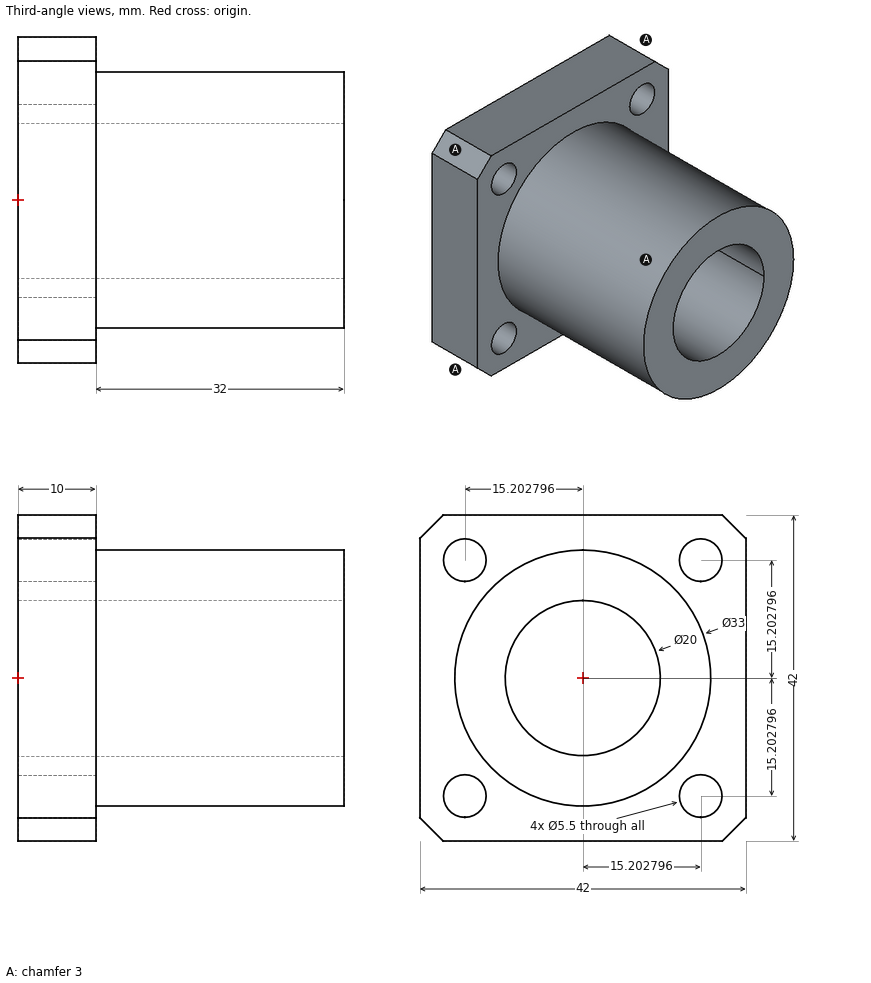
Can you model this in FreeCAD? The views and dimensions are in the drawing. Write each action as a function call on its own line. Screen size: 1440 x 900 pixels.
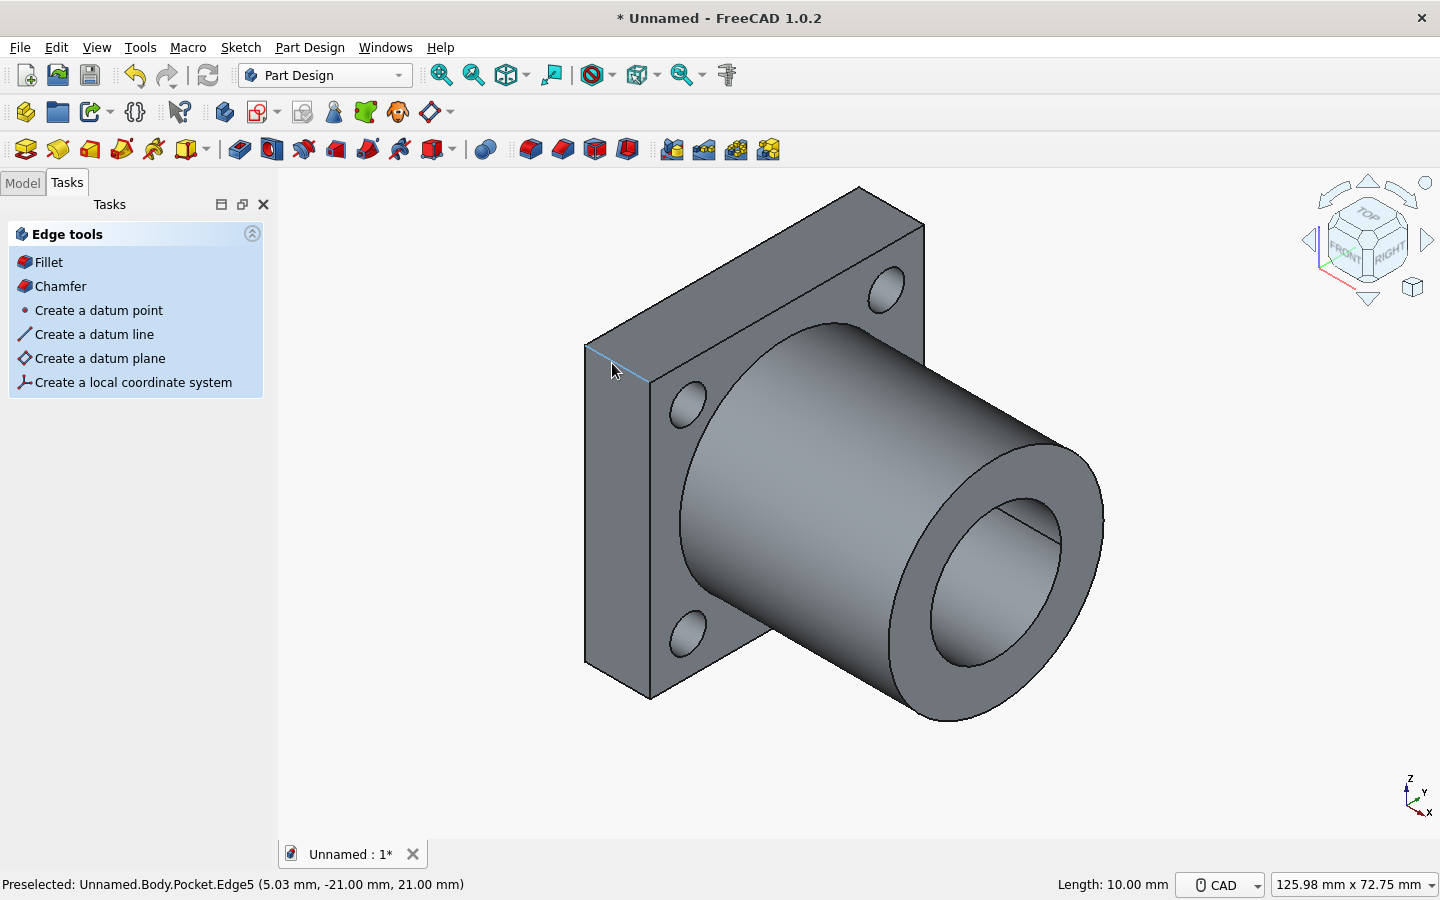
key(2)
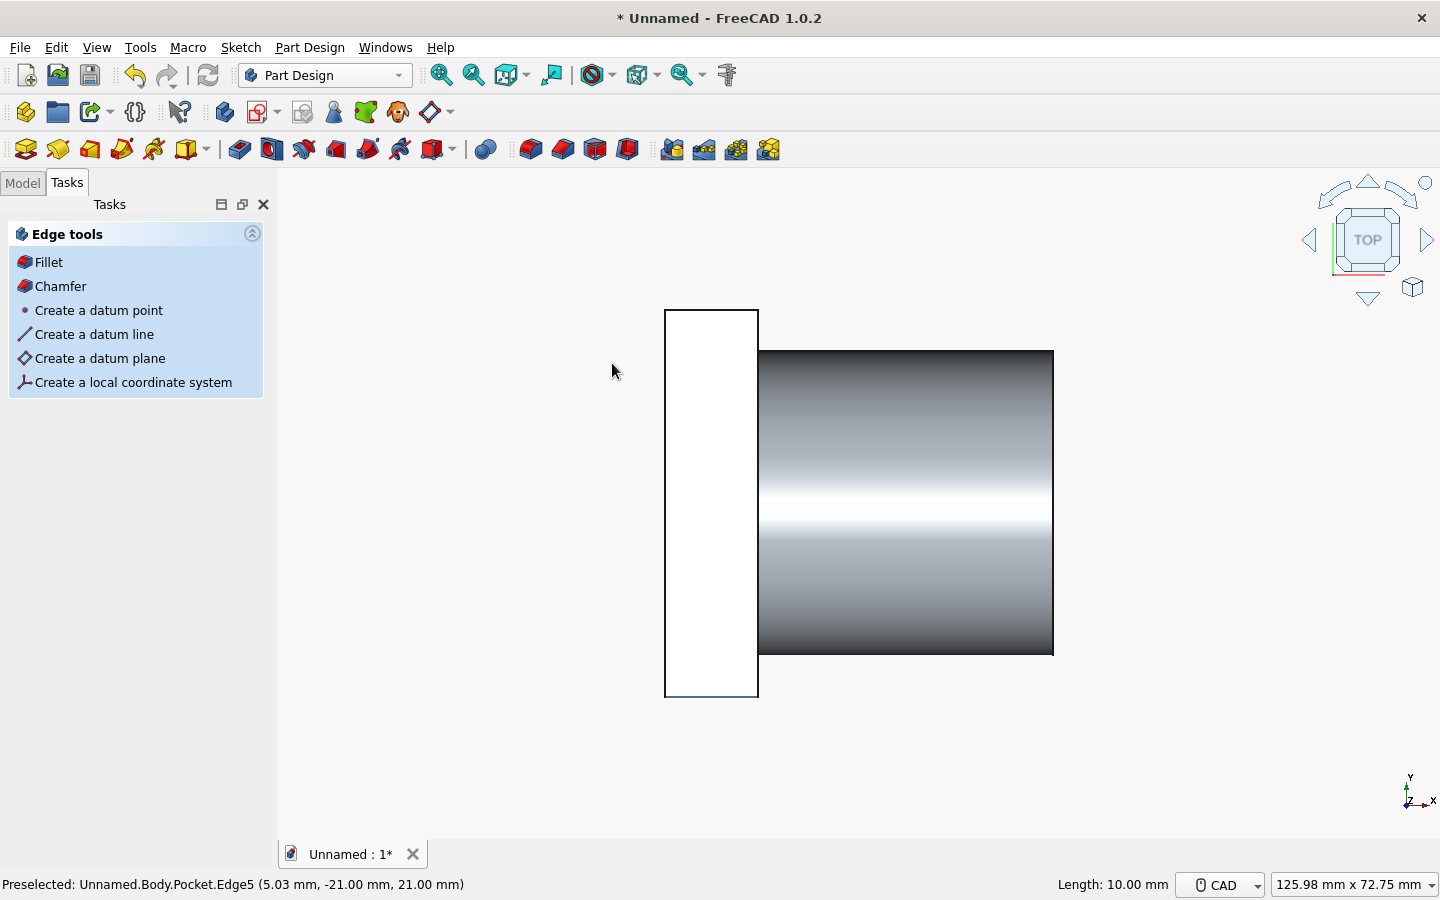
click(711, 309, ctrl)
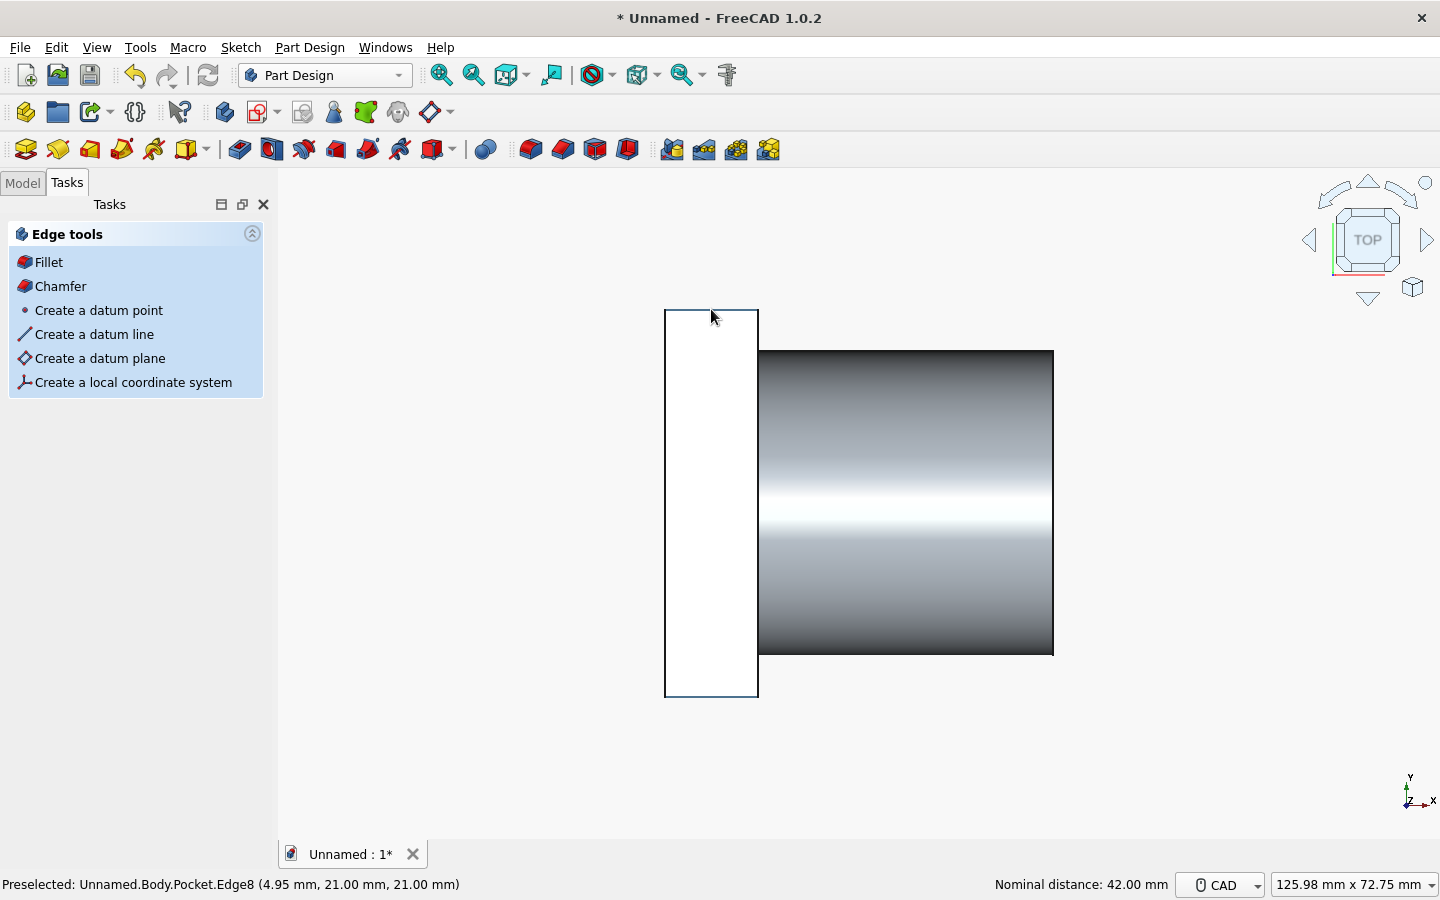
key(1)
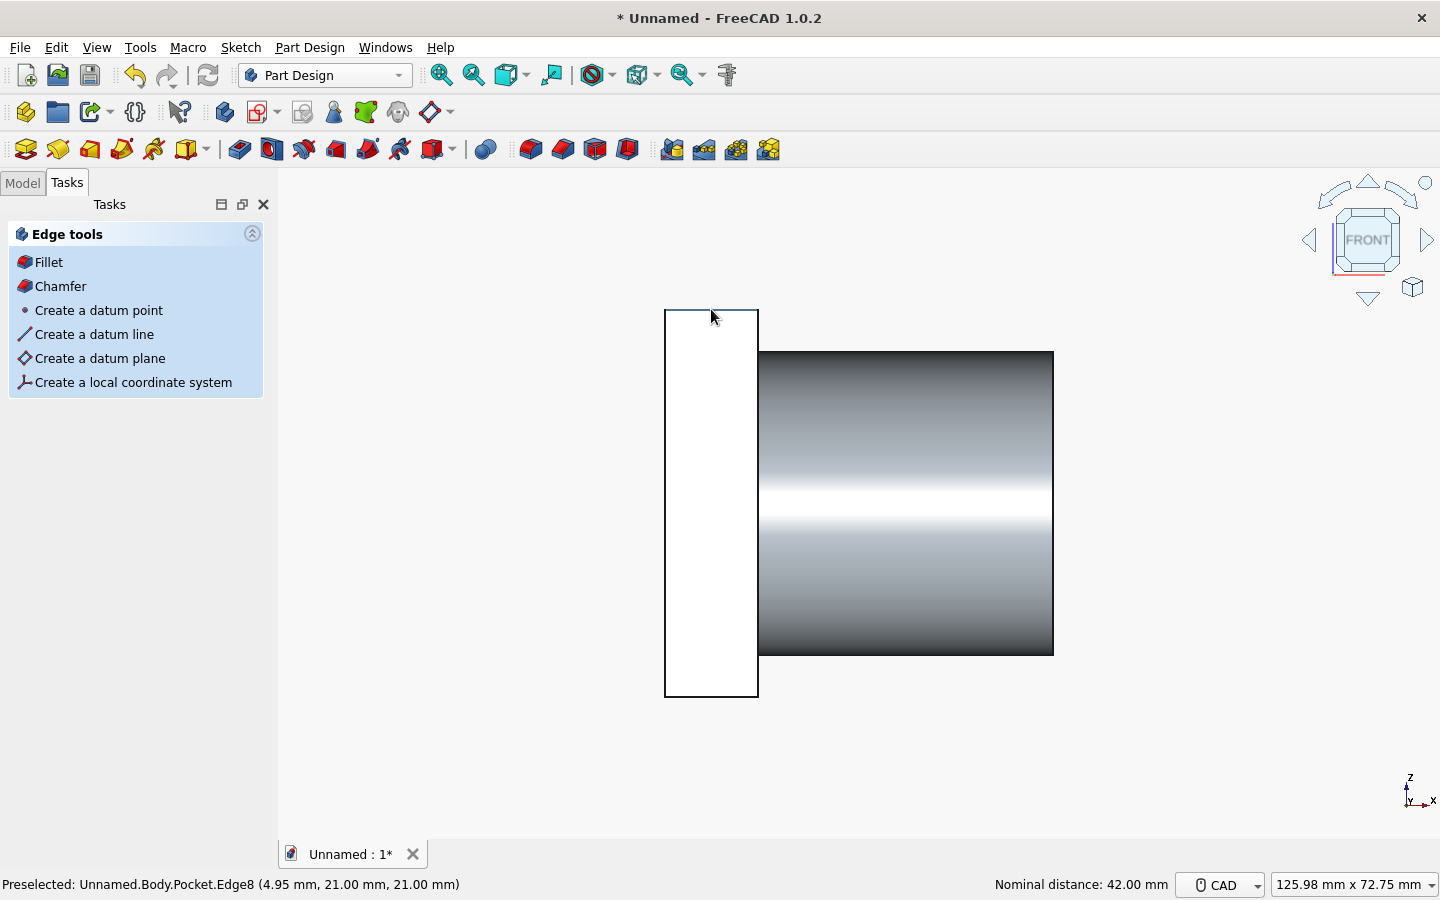
click(711, 696, ctrl)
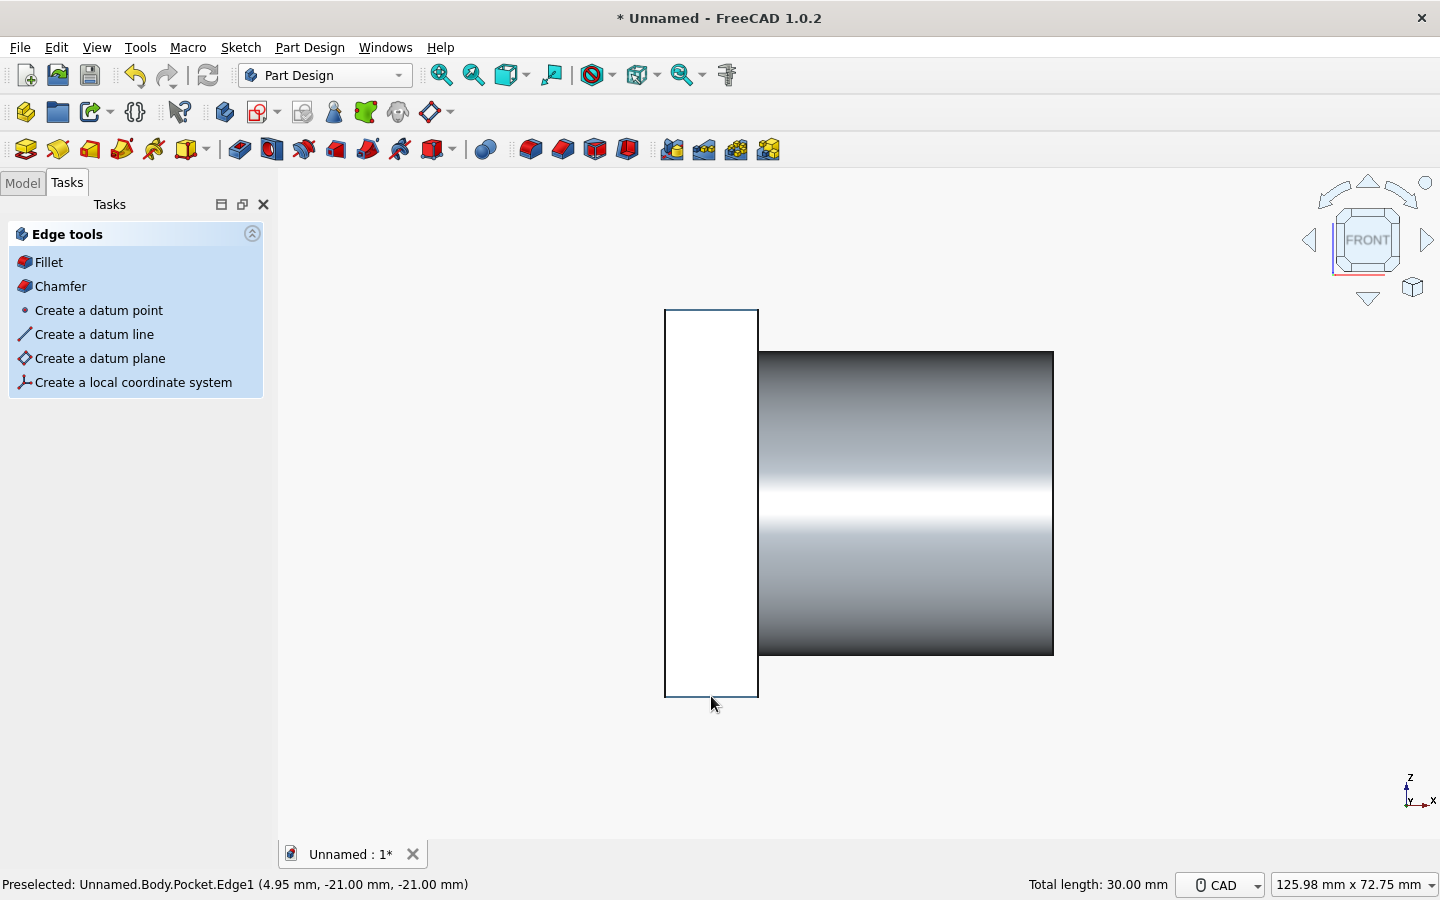
key(3)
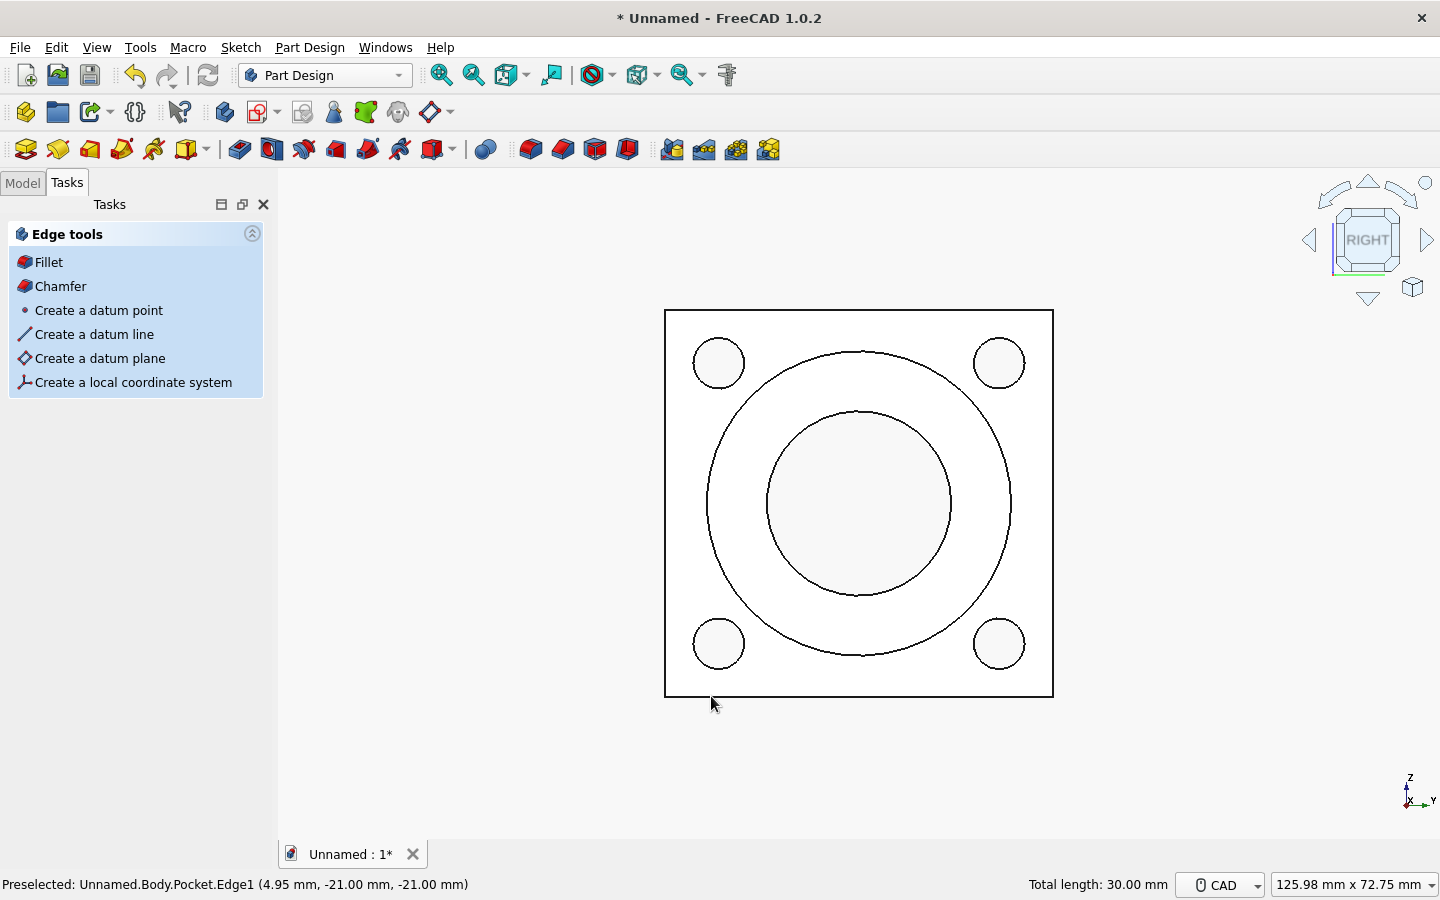
key(5)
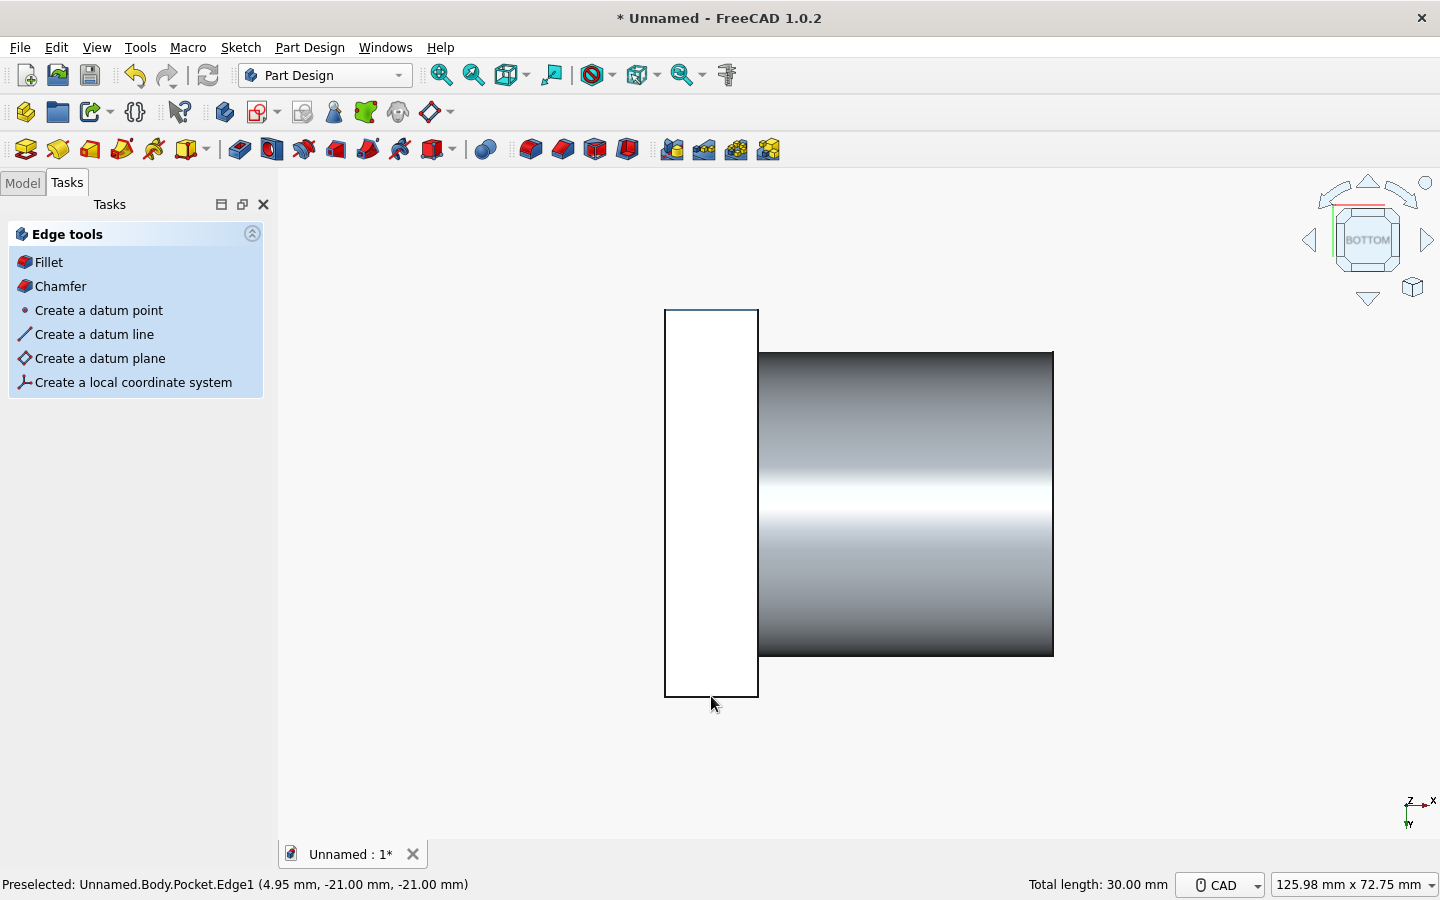
click(711, 696, ctrl)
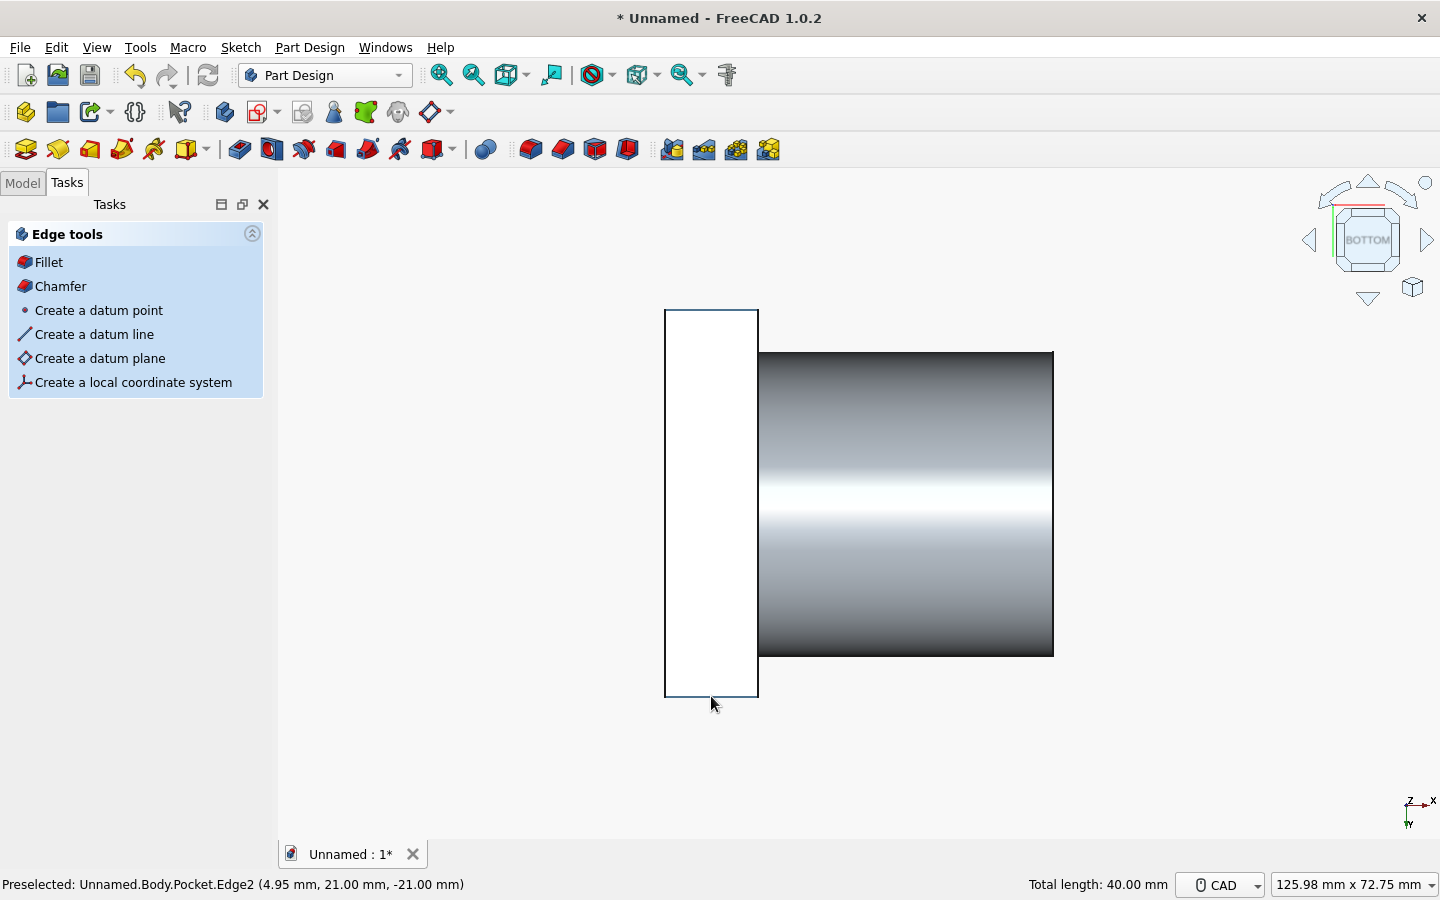
click(564, 150)